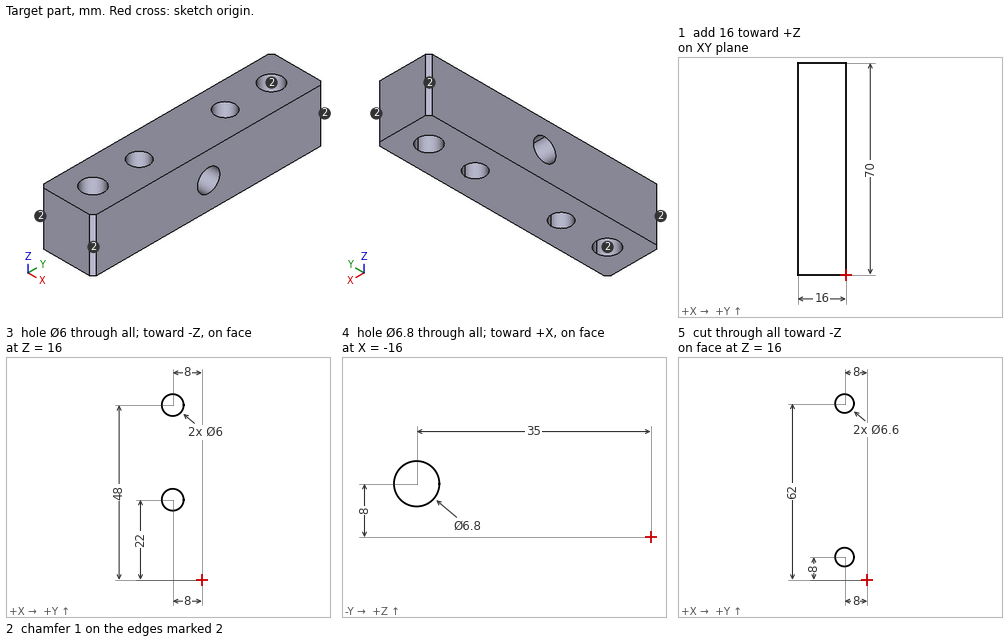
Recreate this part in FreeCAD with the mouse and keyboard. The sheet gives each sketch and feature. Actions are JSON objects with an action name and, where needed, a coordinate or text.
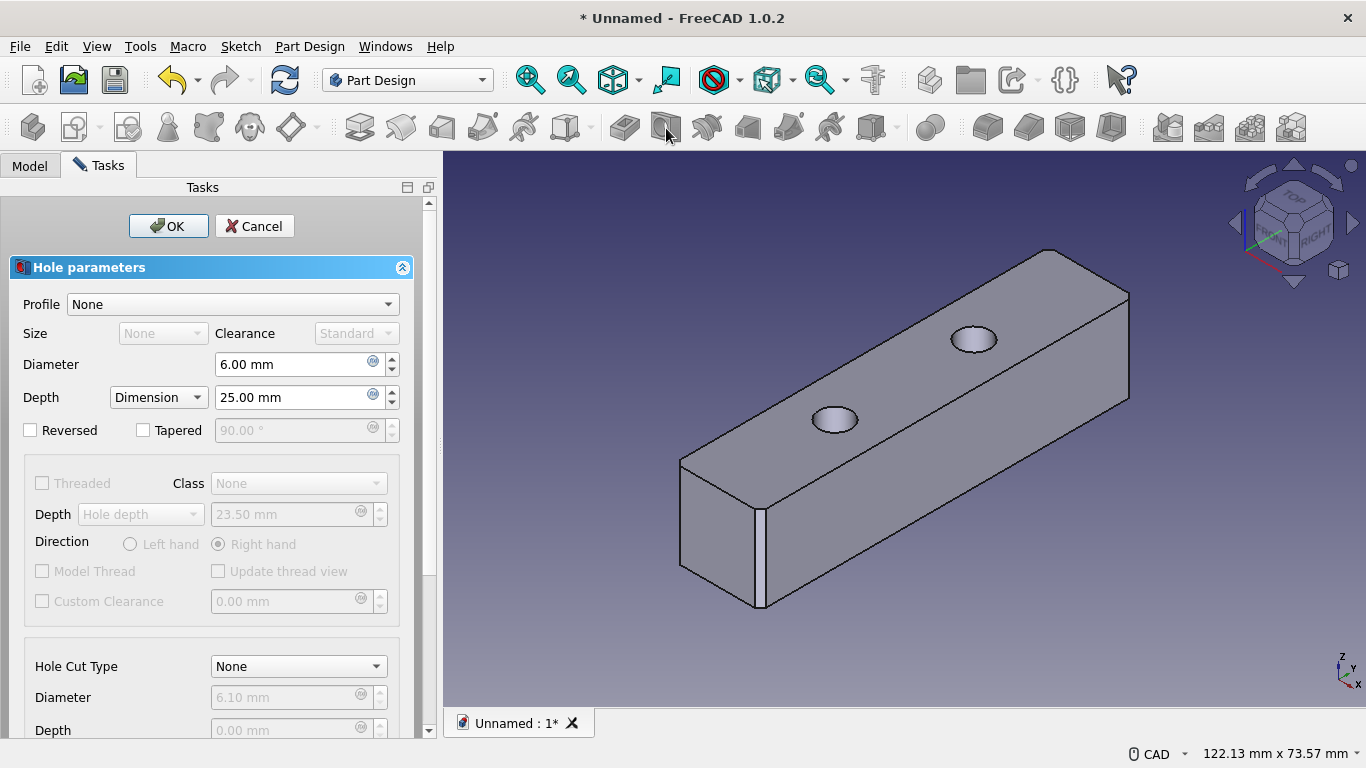
{"action": "triple_click", "coordinate": [300, 364]}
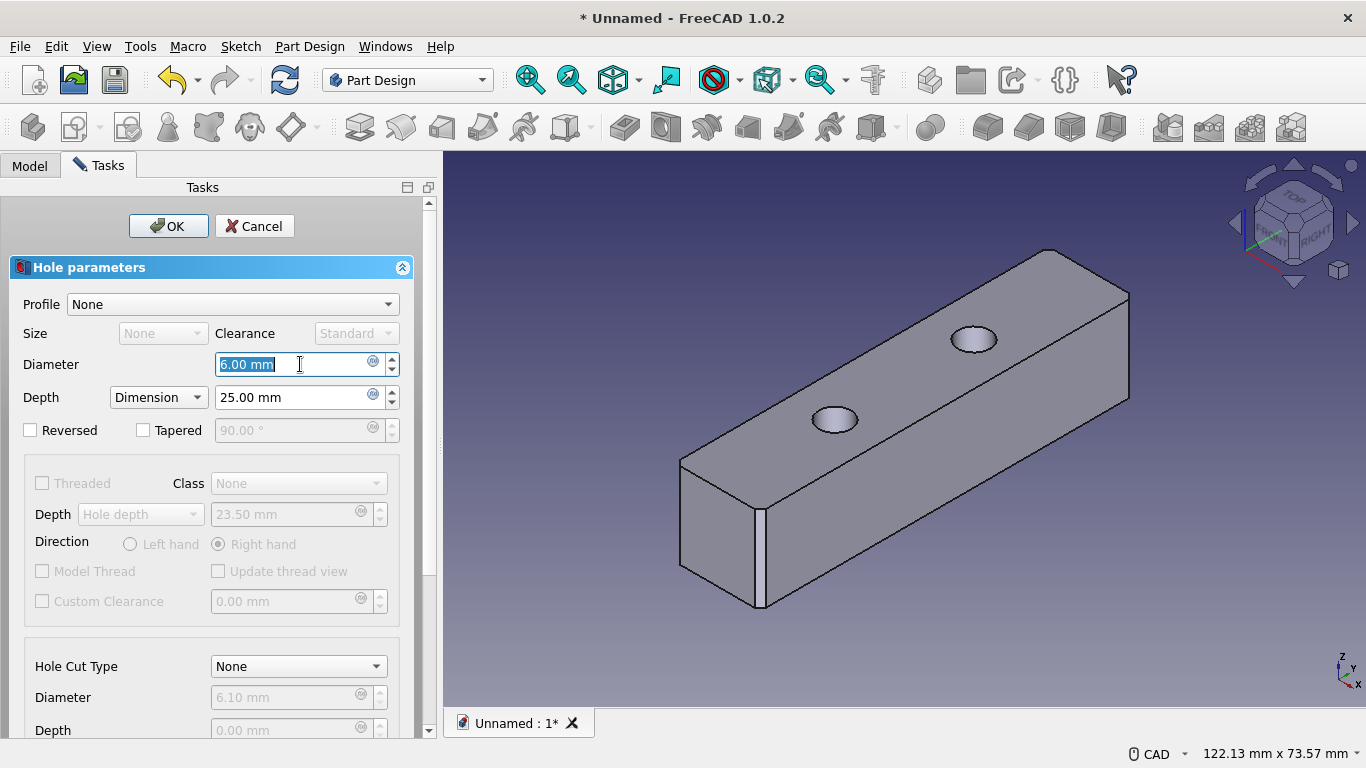
{"action": "type", "text": "6"}
{"action": "key", "text": "Tab"}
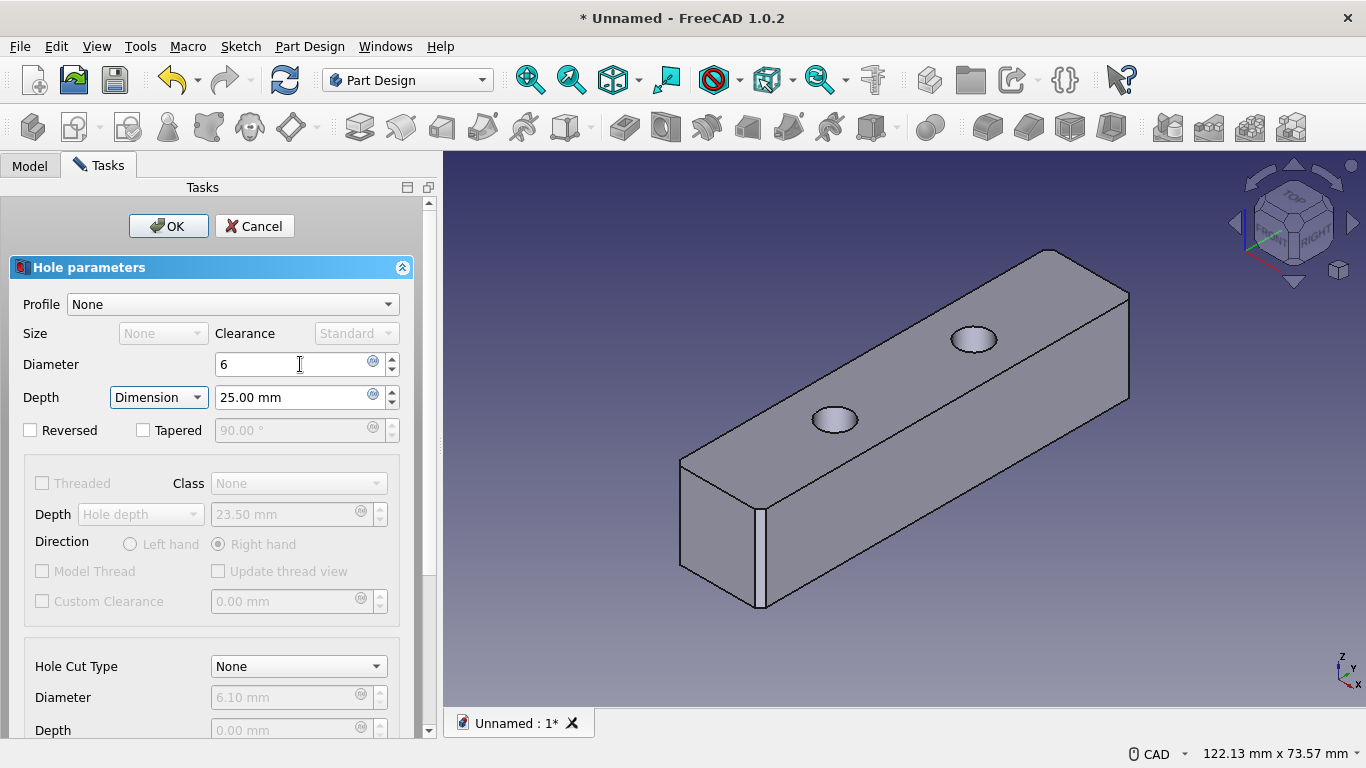
{"action": "left_click", "coordinate": [160, 398]}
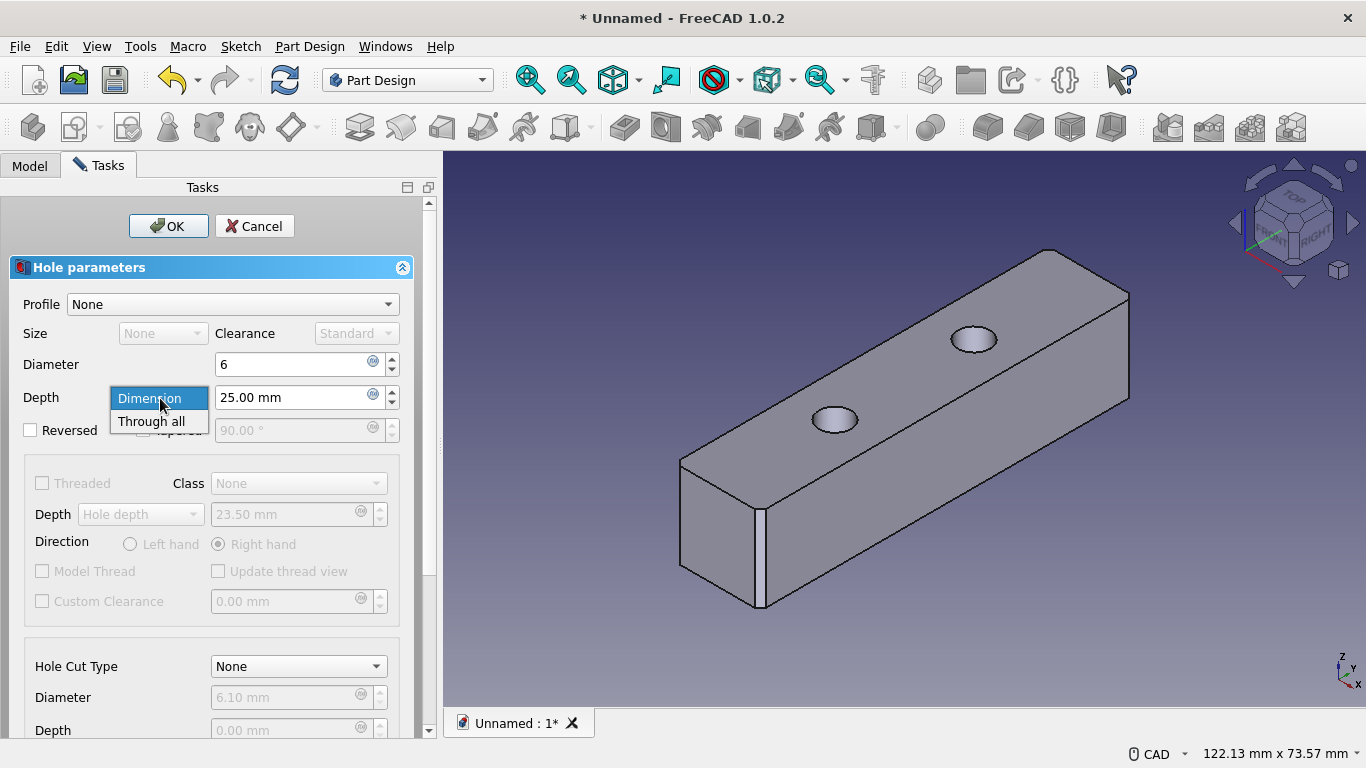
{"action": "left_click", "coordinate": [158, 422]}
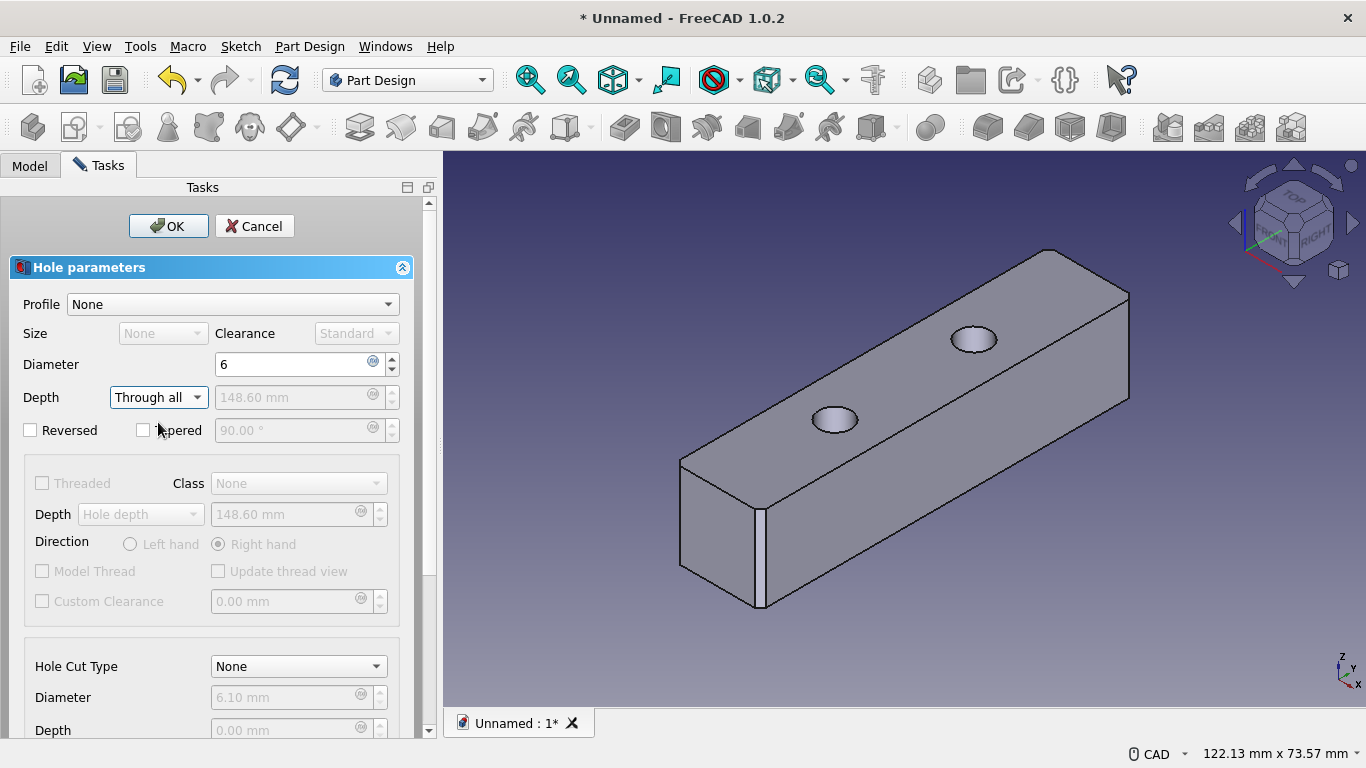
{"action": "left_click", "coordinate": [169, 226]}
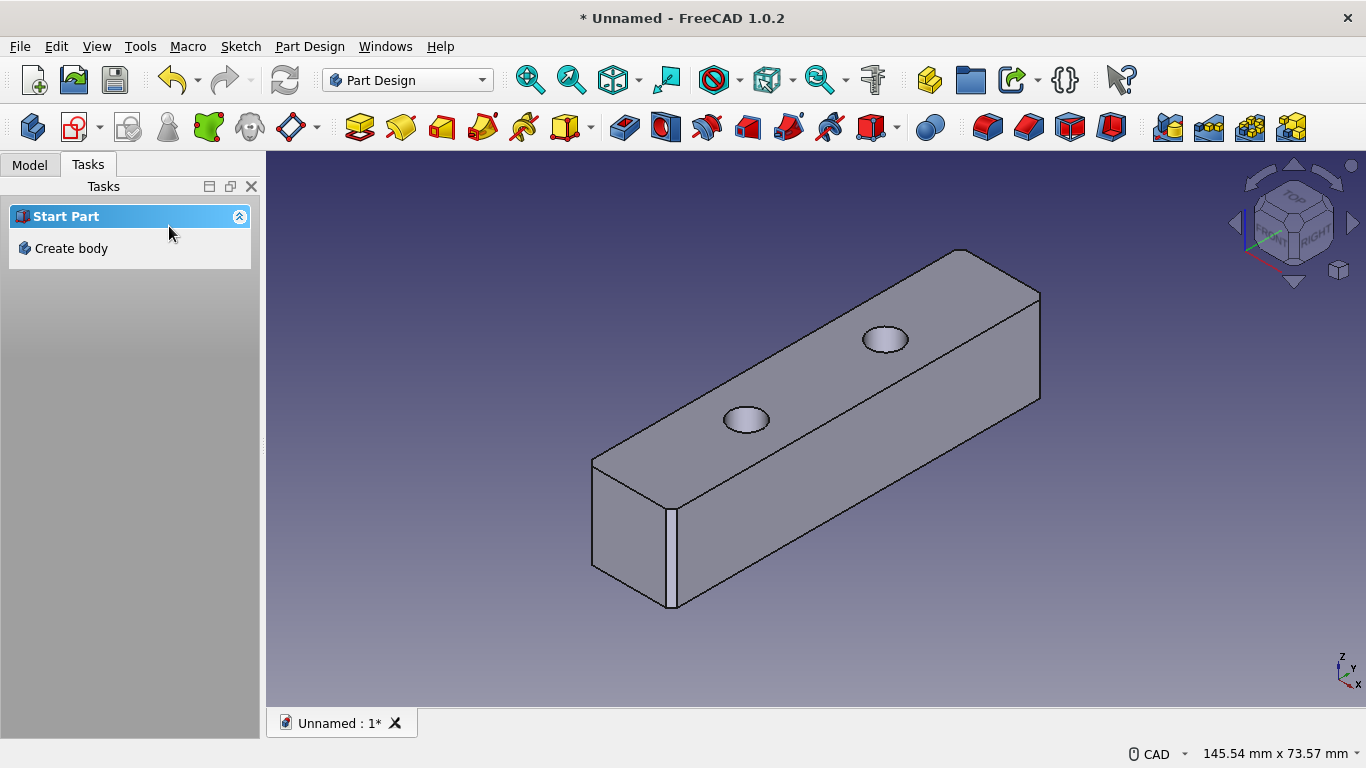
{"action": "key", "text": "6"}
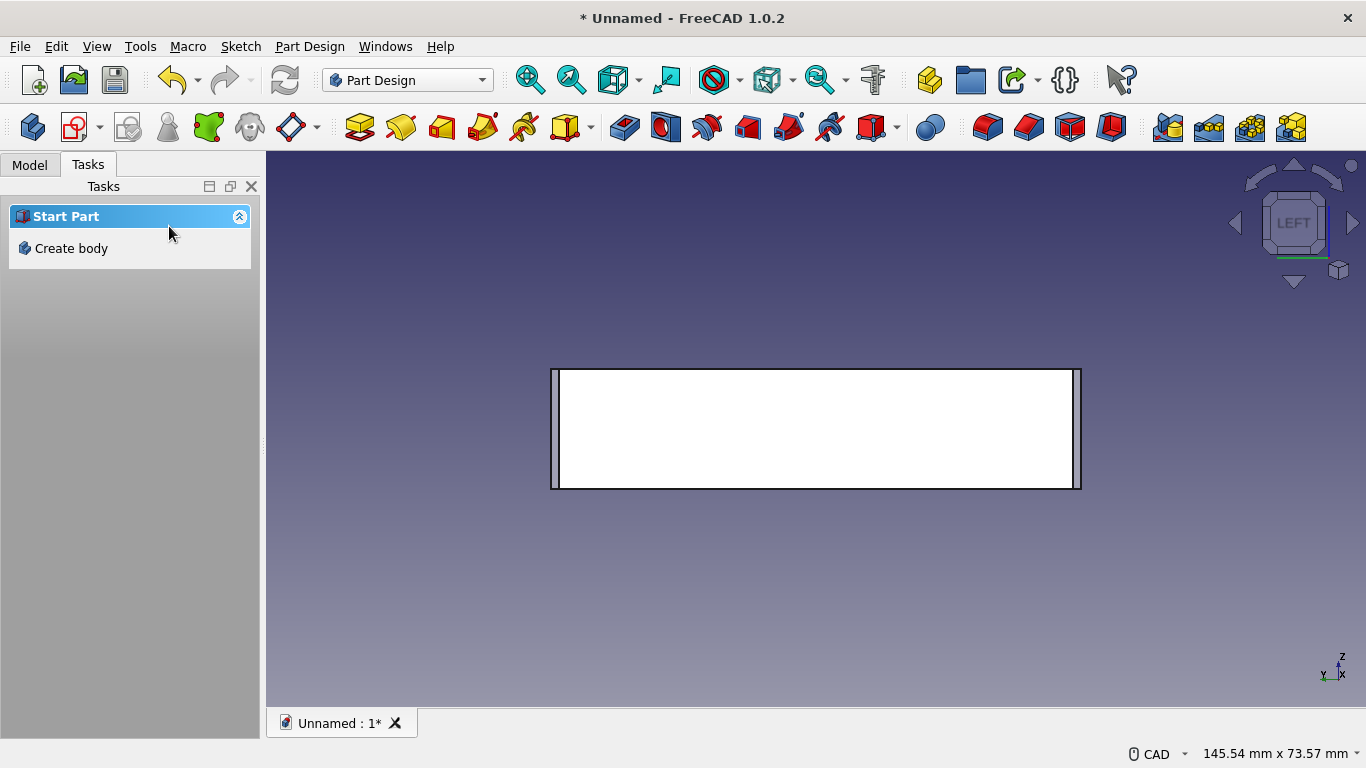
{"action": "left_click", "coordinate": [669, 428]}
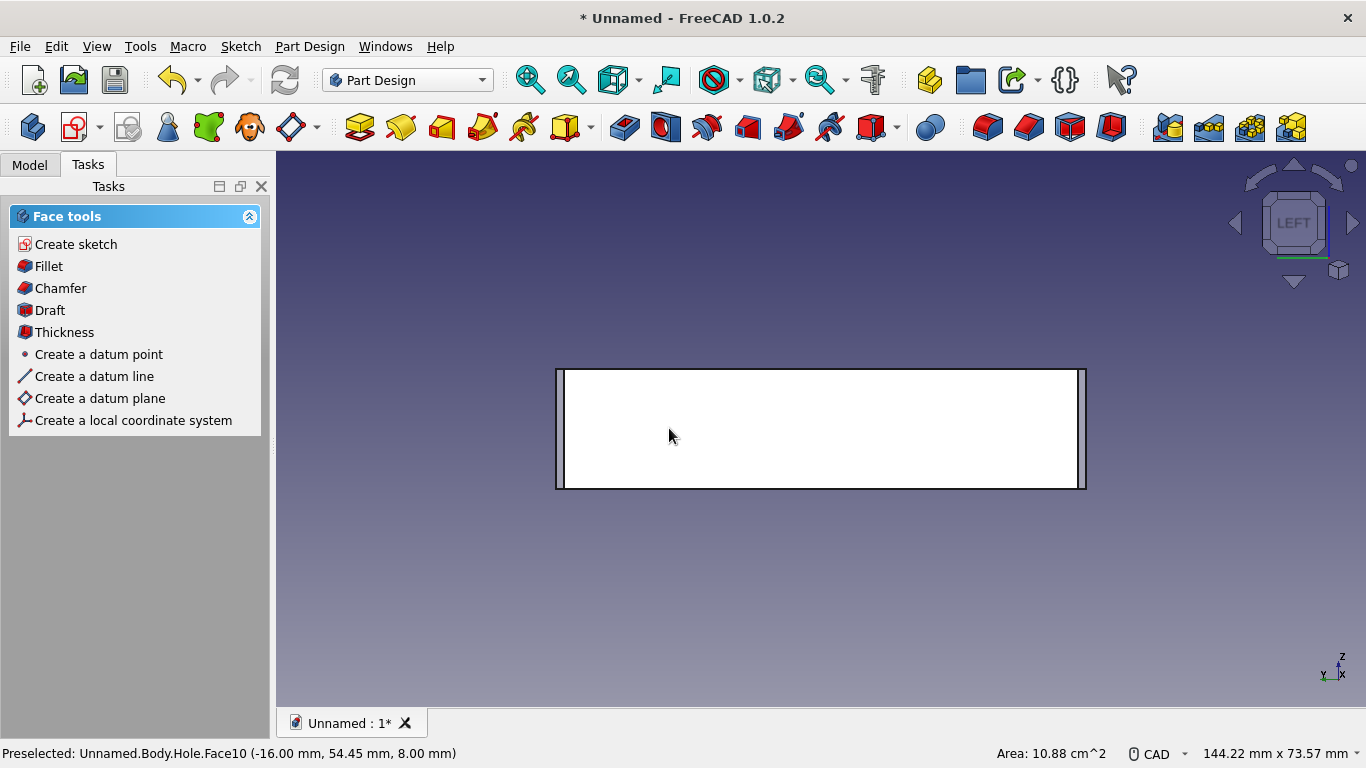
{"action": "left_click", "coordinate": [74, 128]}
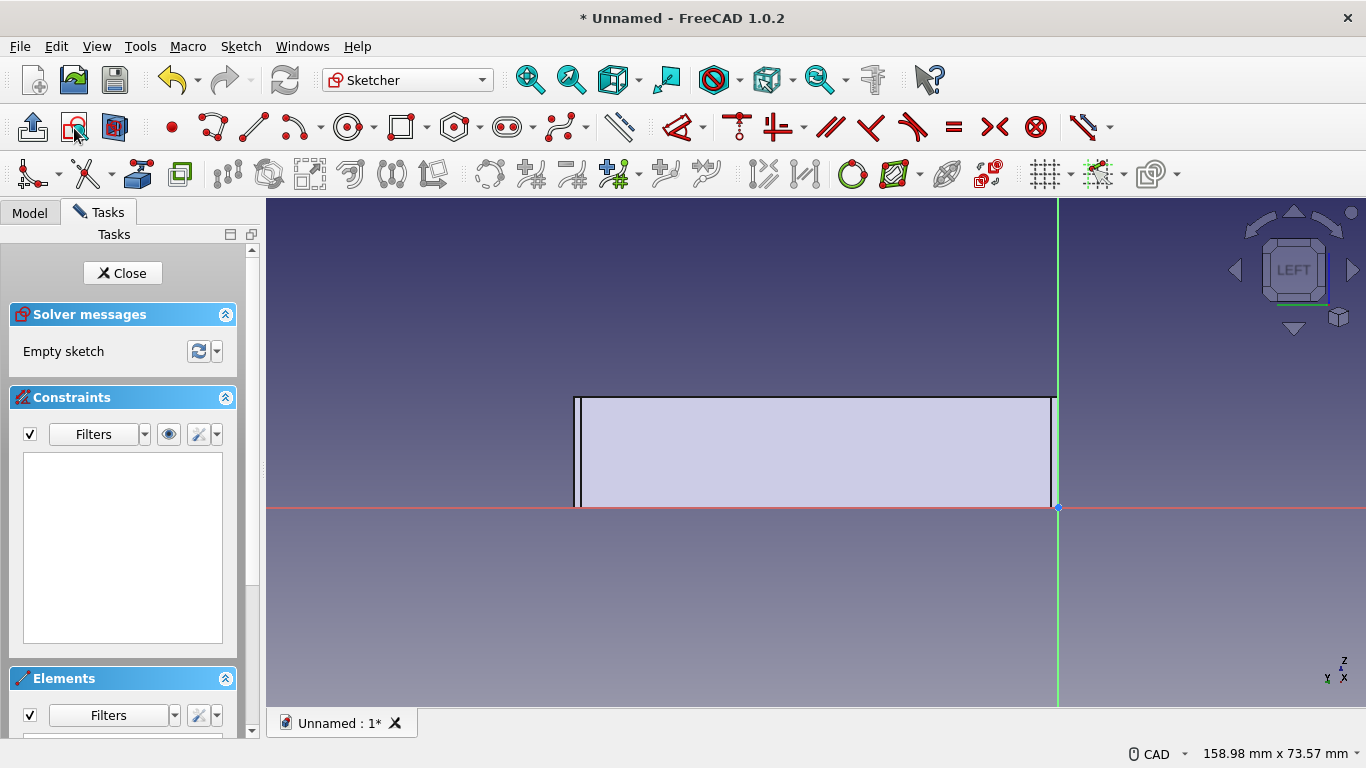
{"action": "scroll", "coordinate": [827, 452], "scroll_direction": "up", "scroll_amount": 10}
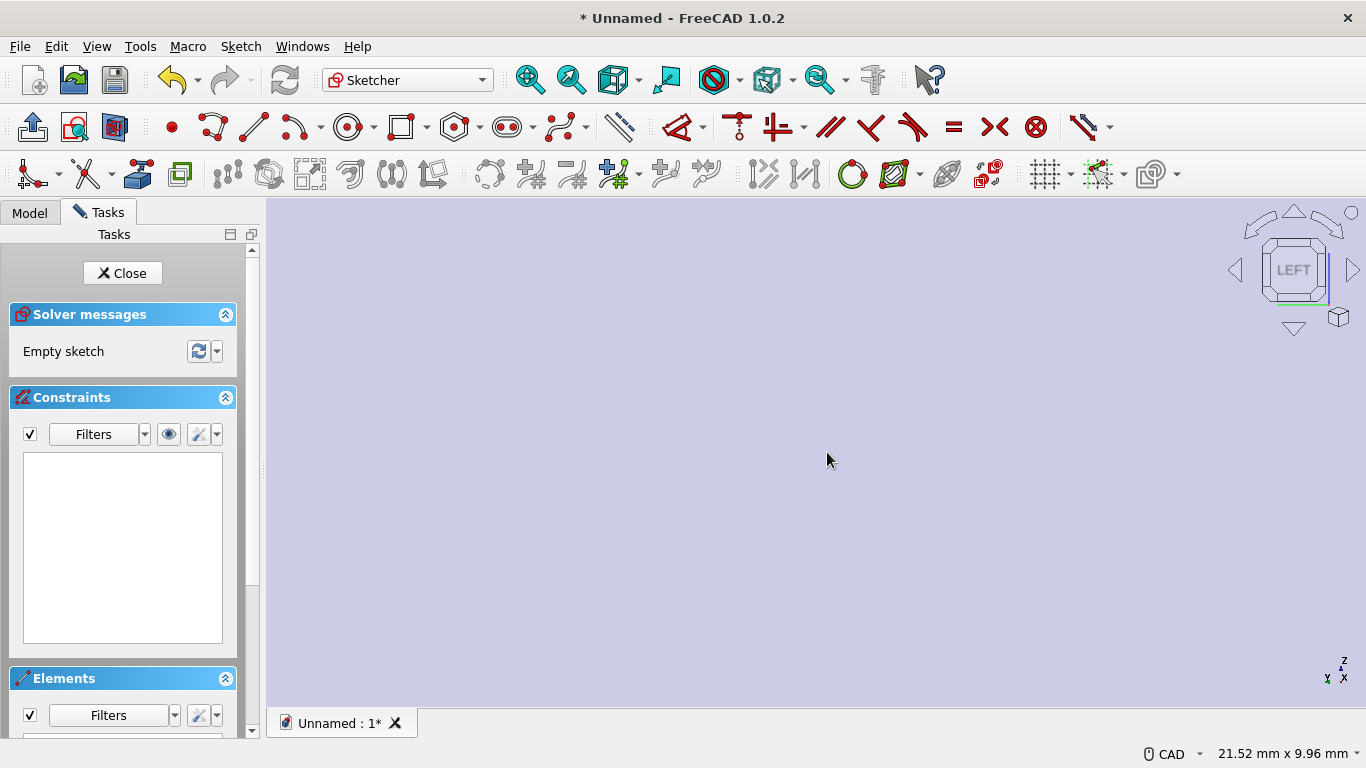
{"action": "left_click", "coordinate": [348, 128]}